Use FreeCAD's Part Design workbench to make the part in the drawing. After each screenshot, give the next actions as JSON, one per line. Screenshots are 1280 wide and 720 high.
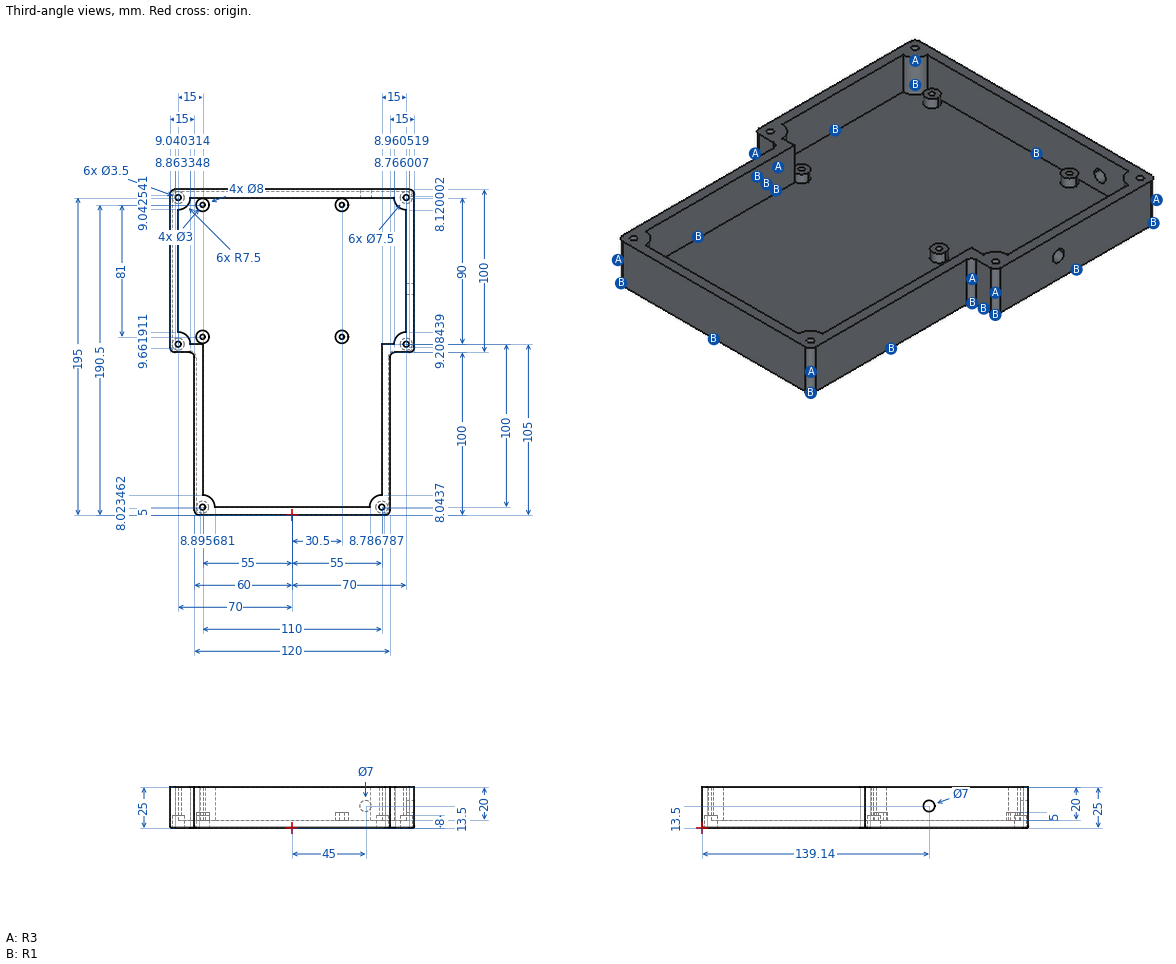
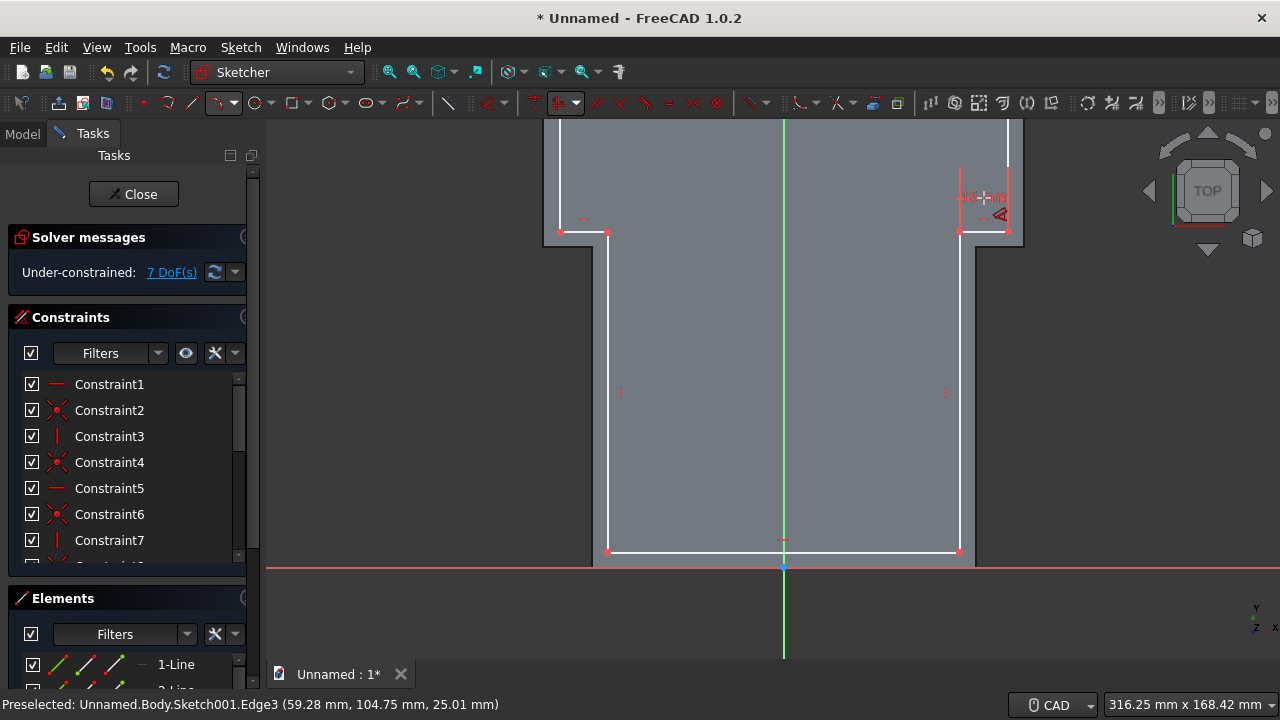
{"action": "left_click", "coordinate": [1008, 174]}
{"action": "left_click", "coordinate": [1042, 170]}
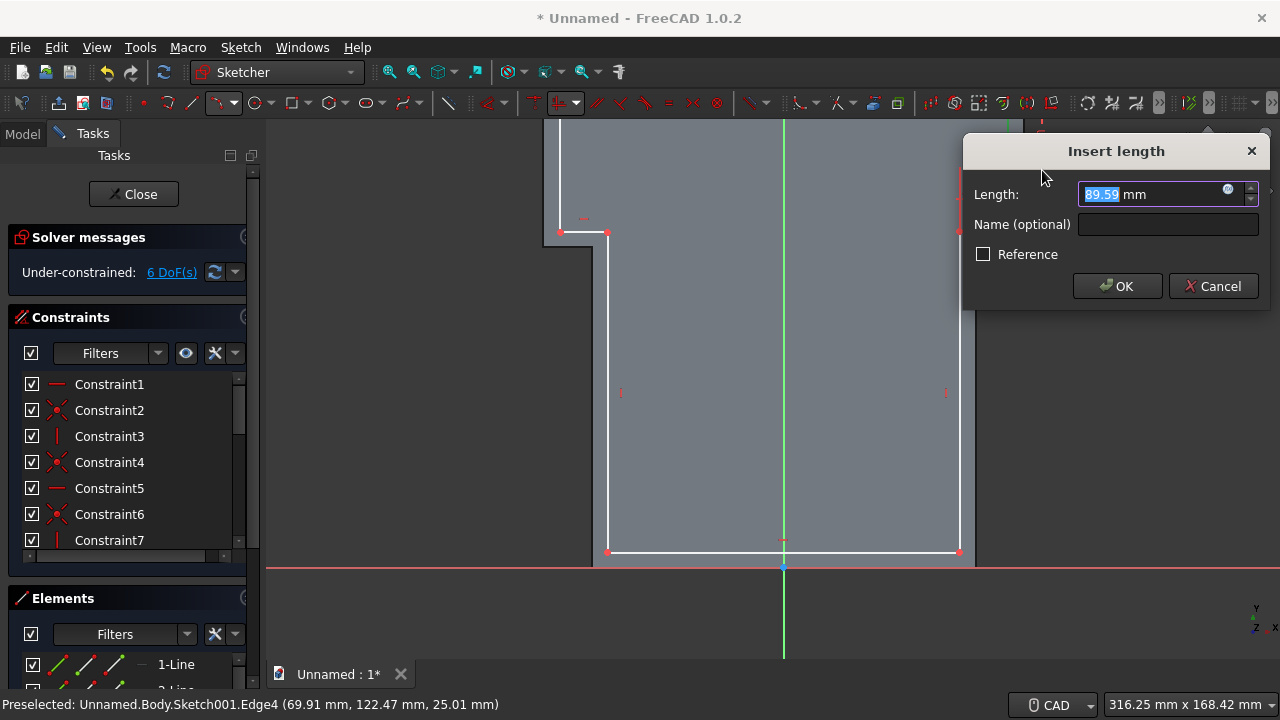
{"action": "type", "text": "90"}
{"action": "key", "text": "Return"}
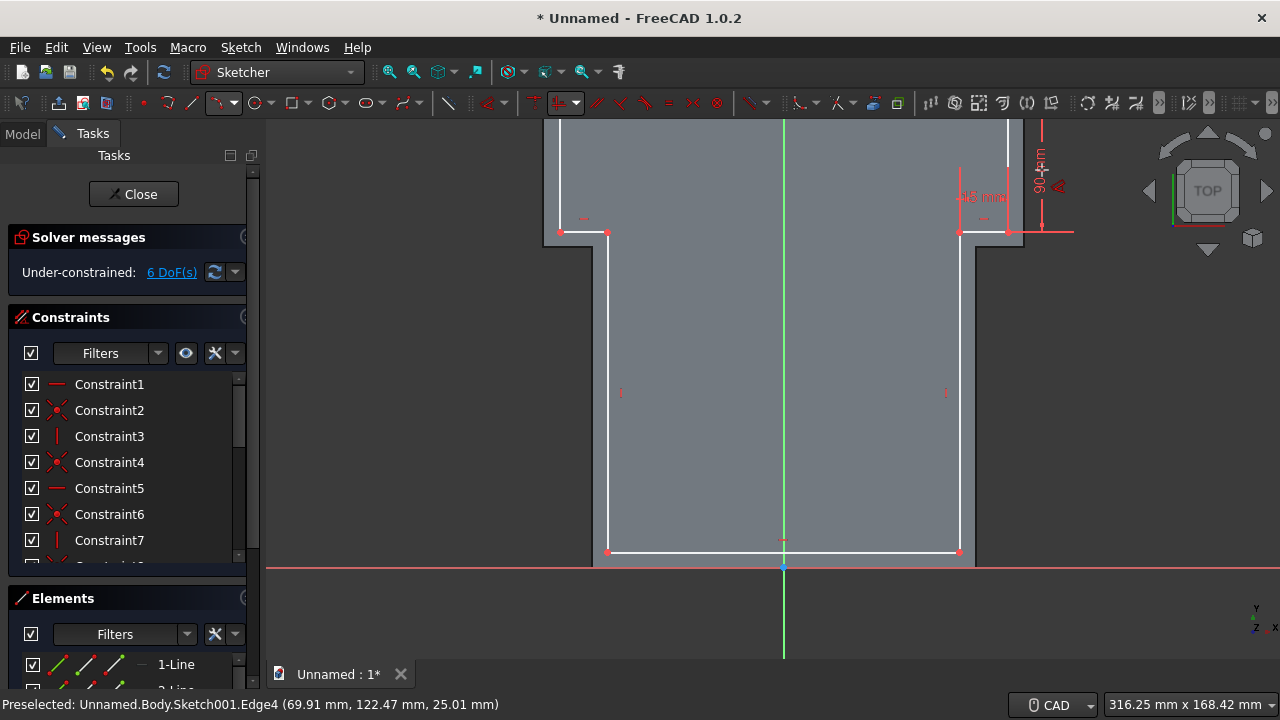
{"action": "left_click", "coordinate": [560, 175]}
{"action": "left_click", "coordinate": [526, 190]}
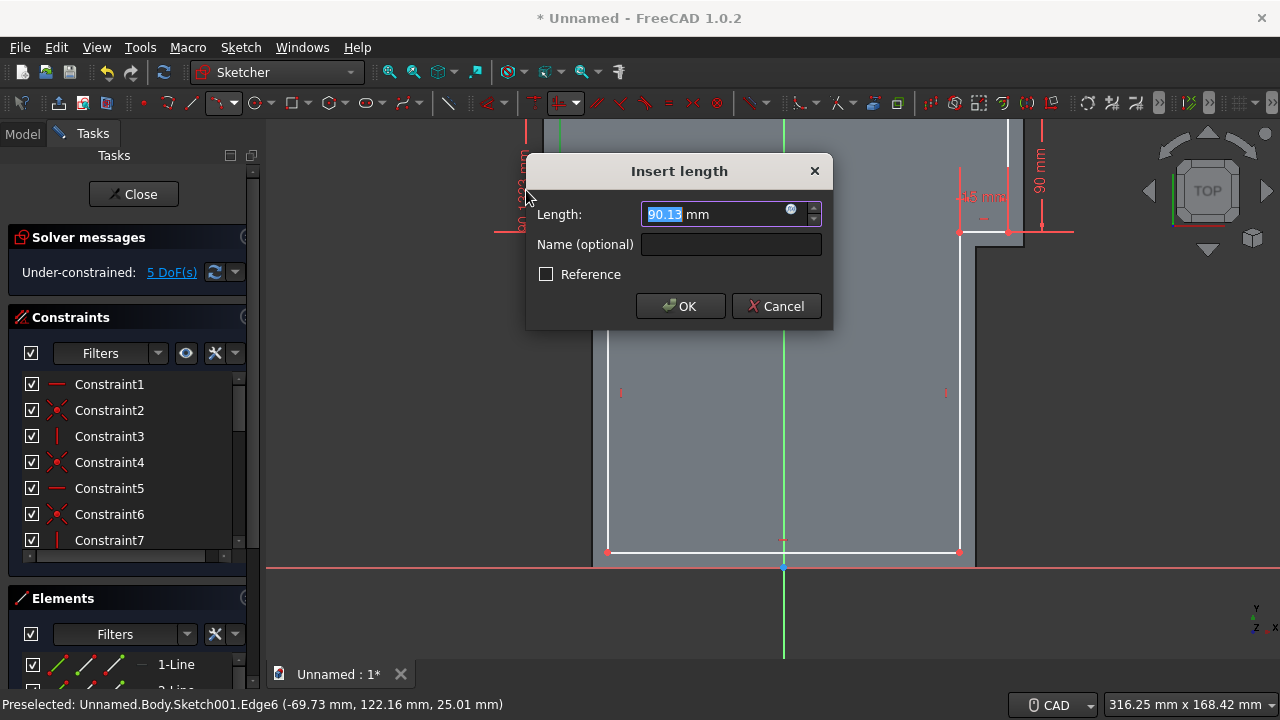
{"action": "type", "text": "90"}
{"action": "key", "text": "Return"}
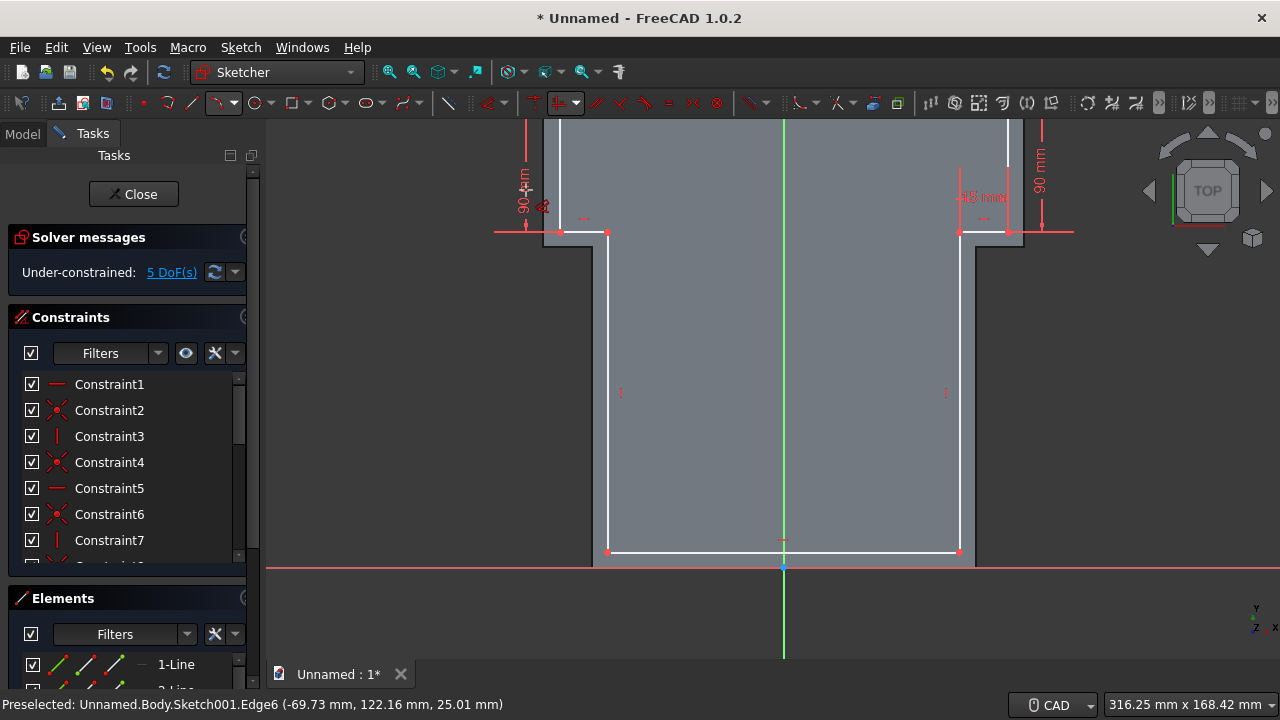
{"action": "left_click", "coordinate": [575, 232]}
{"action": "left_click", "coordinate": [601, 198]}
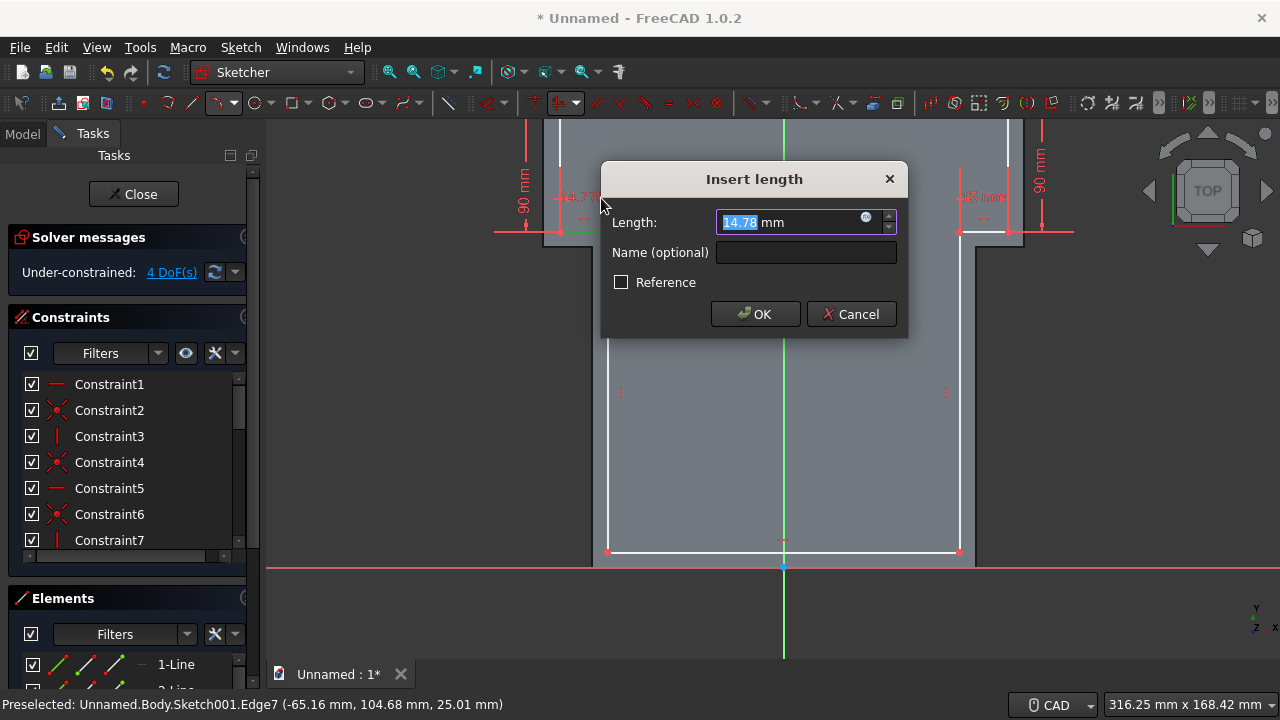
{"action": "type", "text": "15"}
{"action": "key", "text": "Return"}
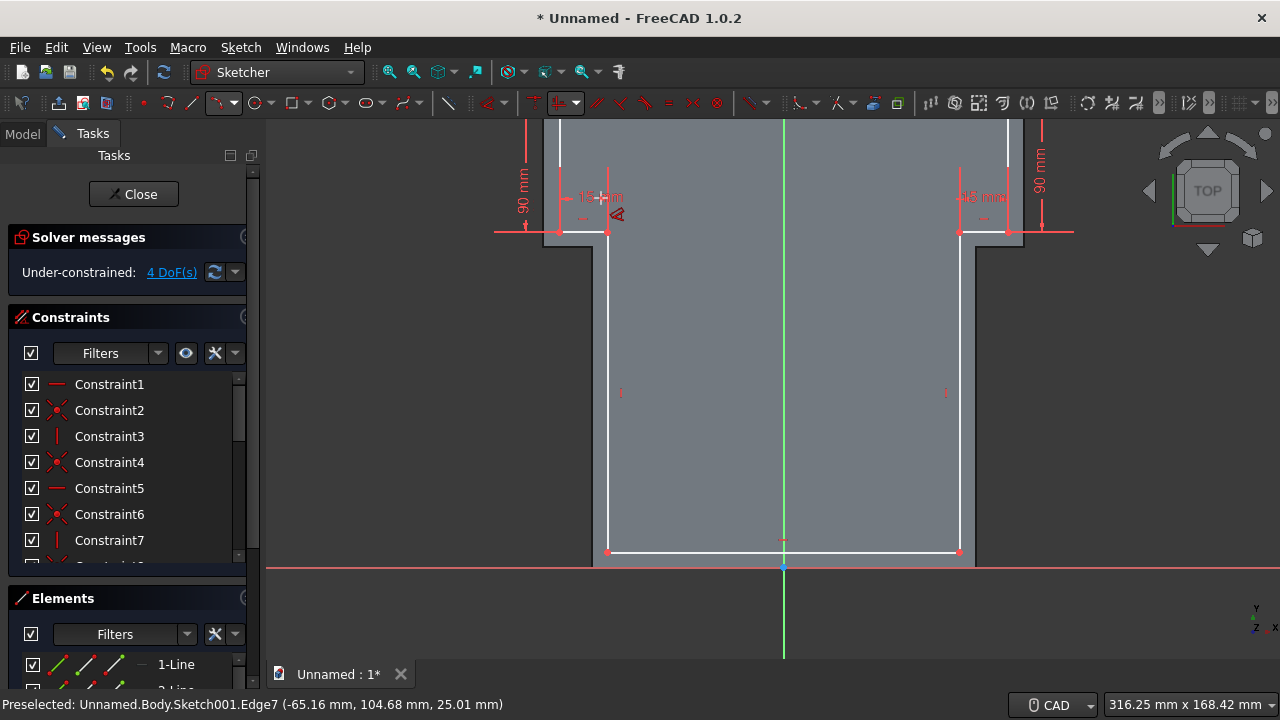
{"action": "scroll", "coordinate": [608, 553], "scroll_direction": "up", "scroll_amount": 5}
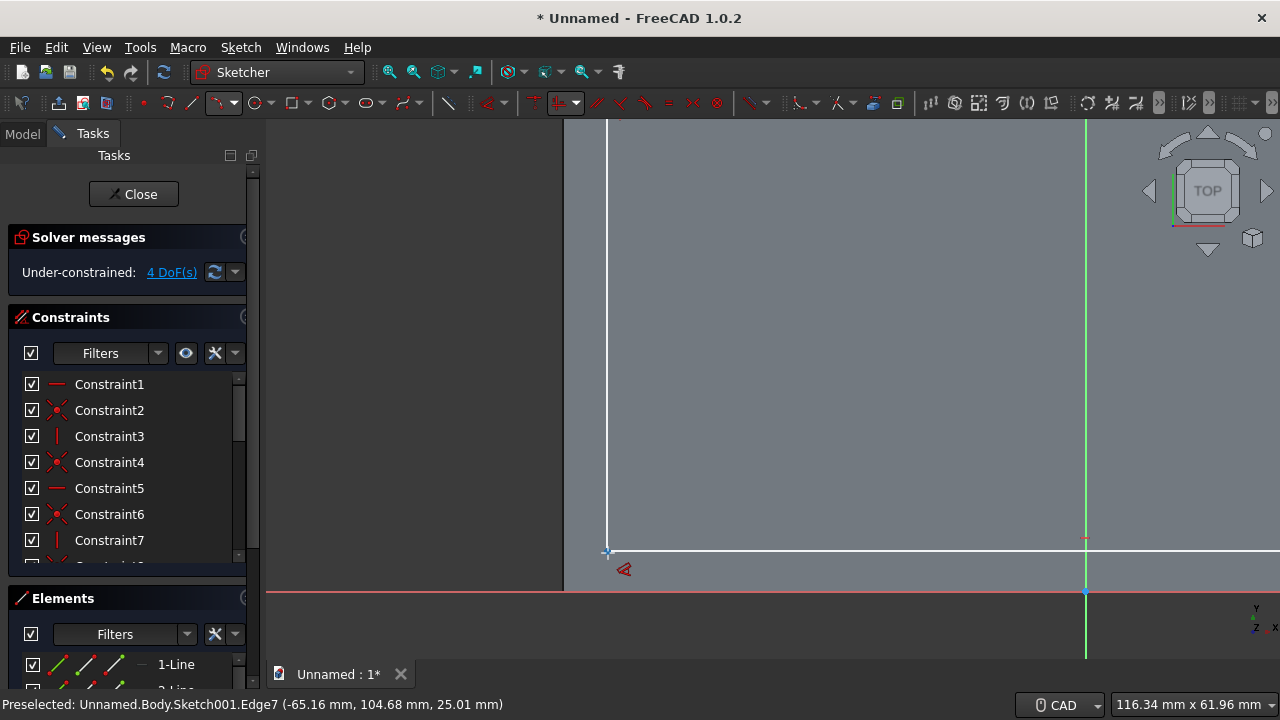
{"action": "left_click", "coordinate": [607, 551]}
{"action": "left_click", "coordinate": [573, 571]}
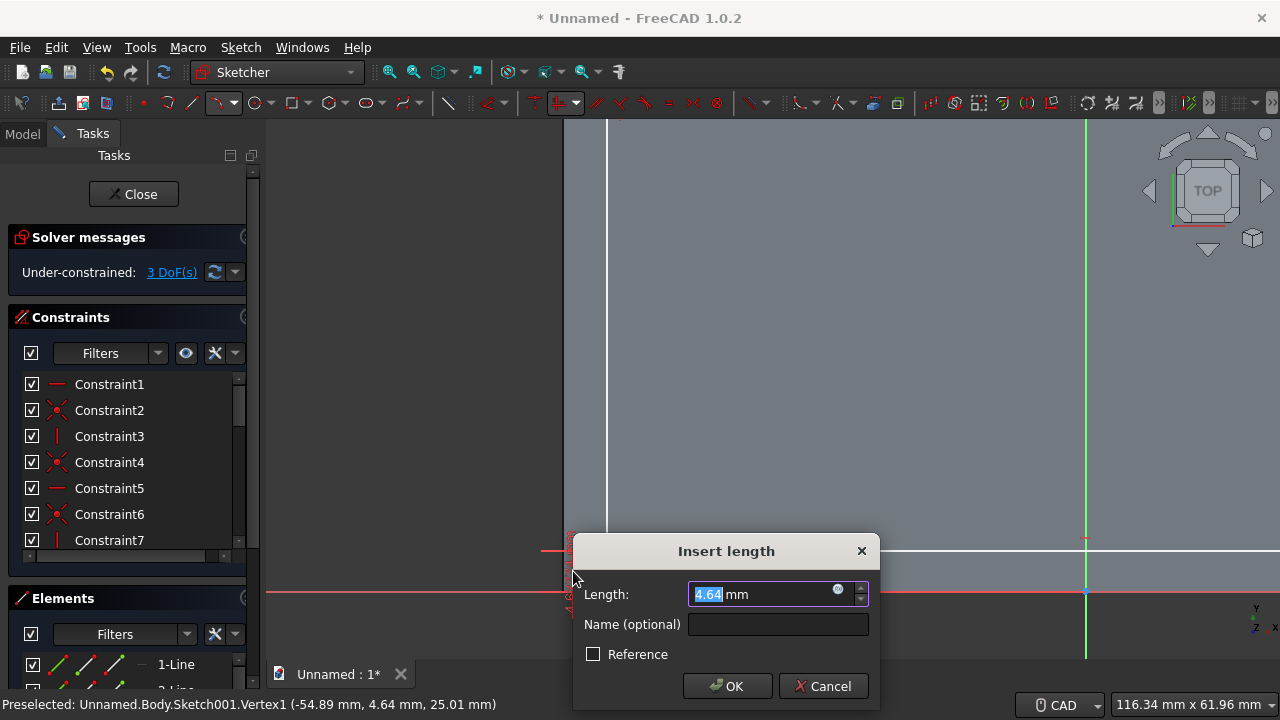
{"action": "type", "text": "5"}
{"action": "key", "text": "Return"}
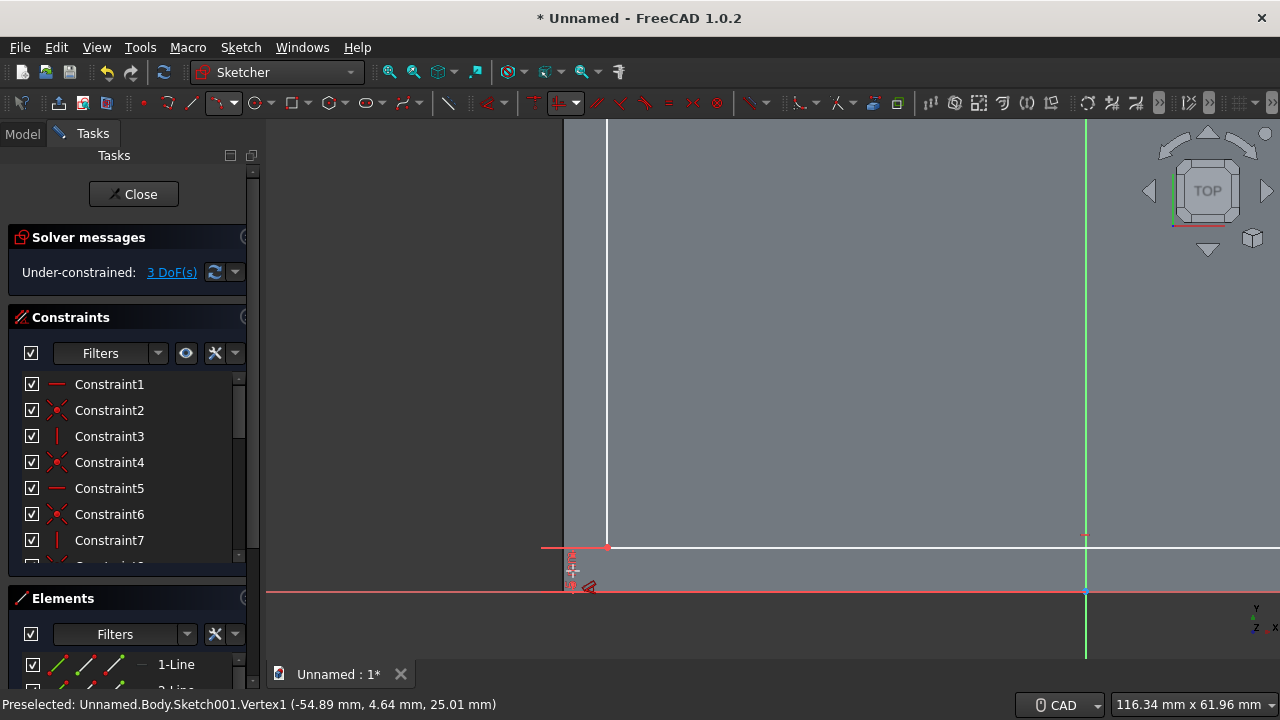
{"action": "scroll", "coordinate": [608, 553], "scroll_direction": "down", "scroll_amount": 8}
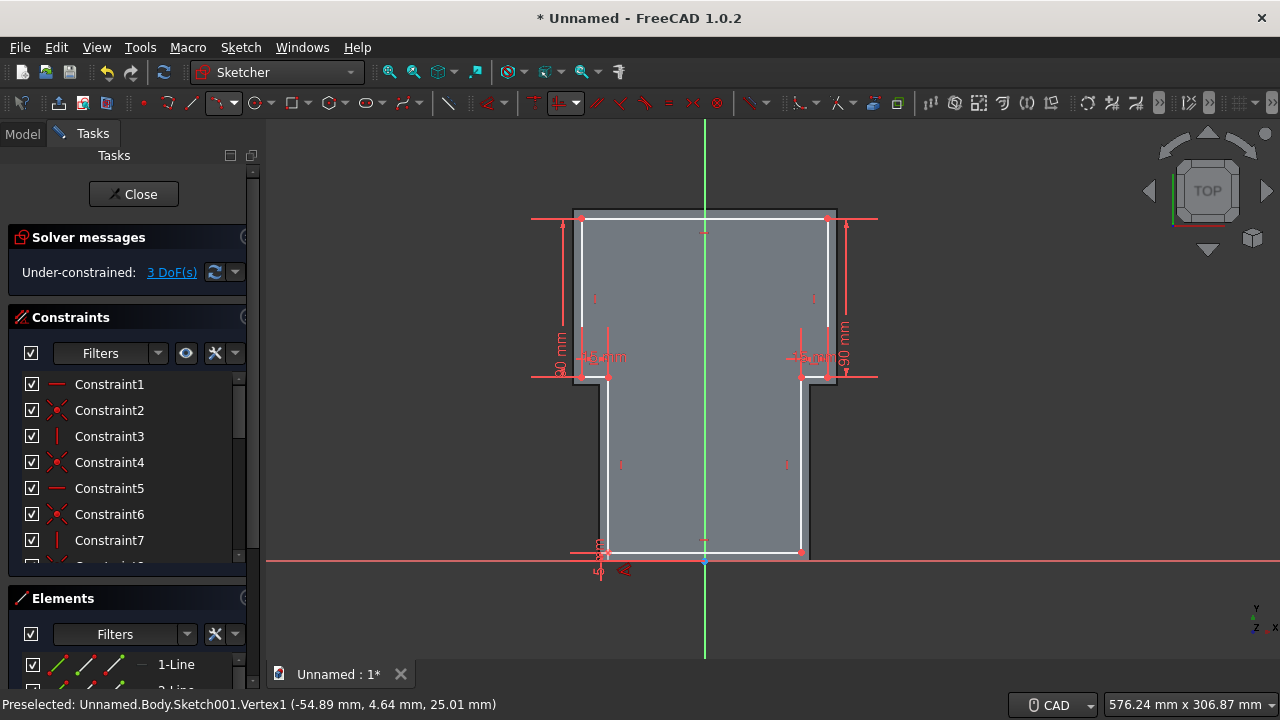
{"action": "scroll", "coordinate": [666, 553], "scroll_direction": "up", "scroll_amount": 3}